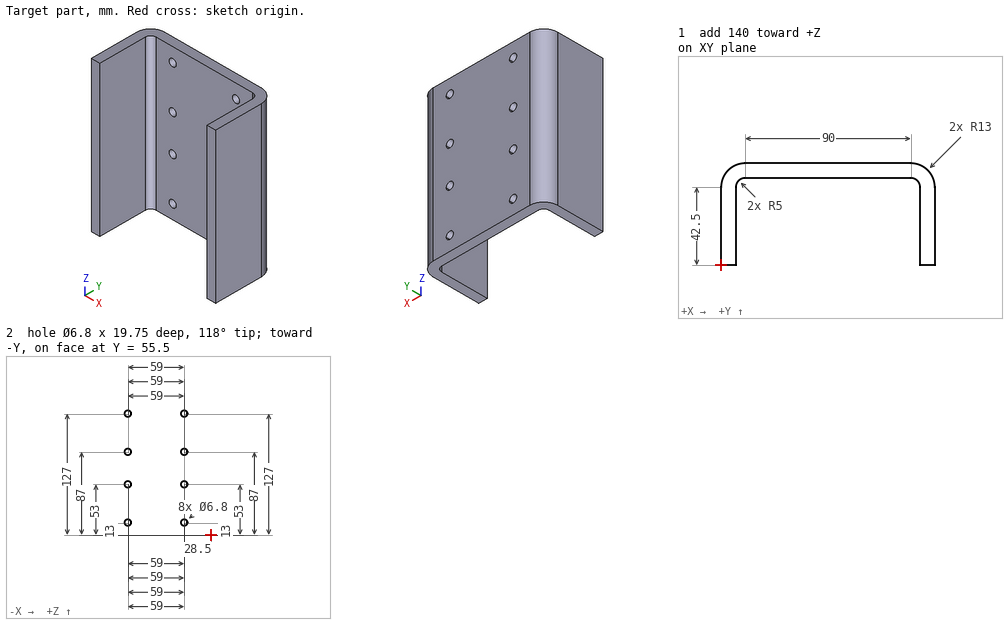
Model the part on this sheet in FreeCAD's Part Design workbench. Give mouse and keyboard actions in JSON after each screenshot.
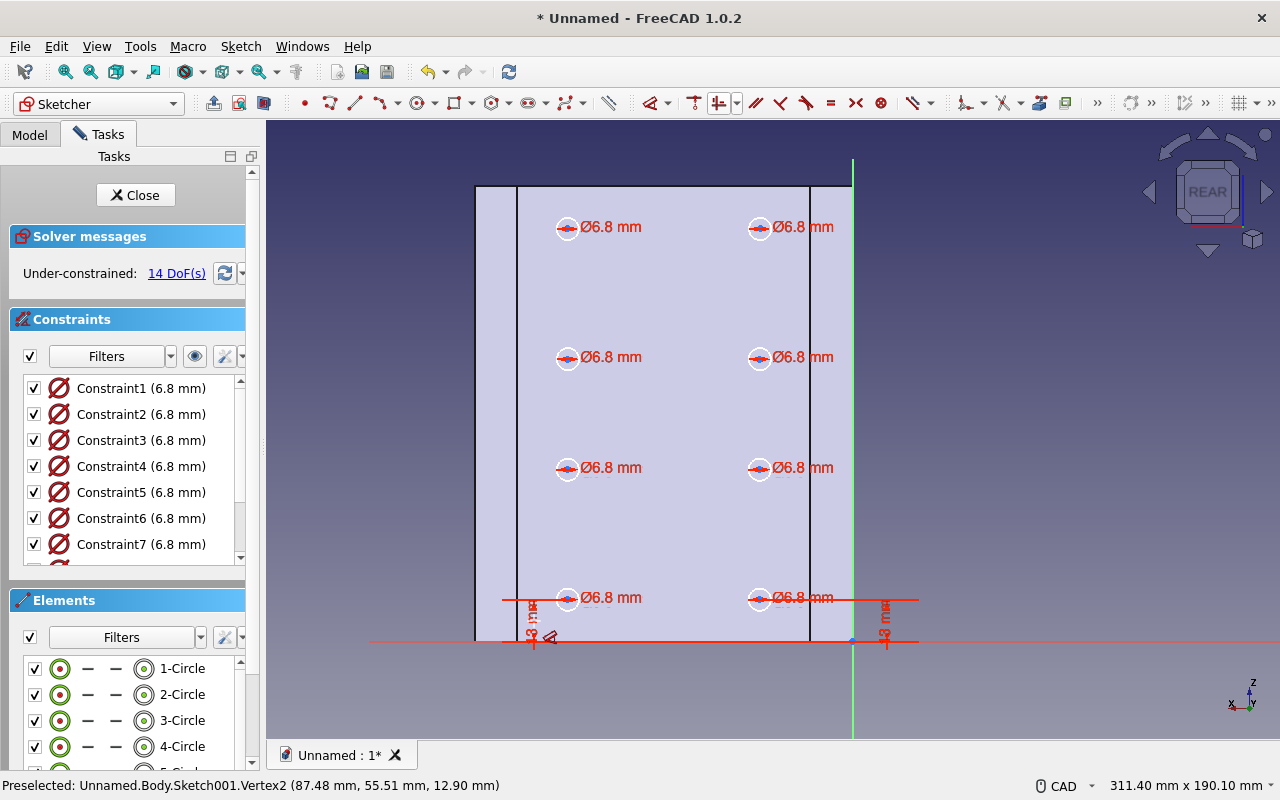
{"action": "left_click", "coordinate": [568, 470]}
{"action": "left_click", "coordinate": [887, 556]}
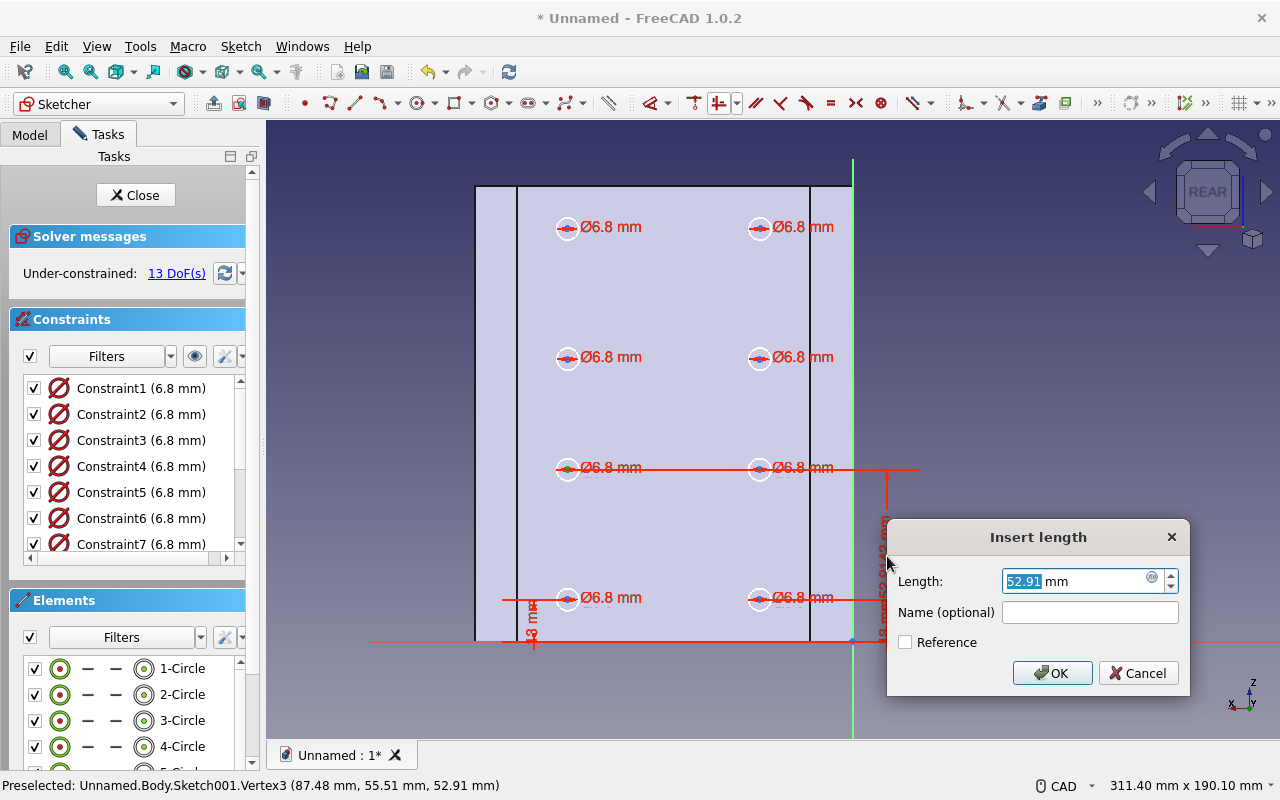
{"action": "type", "text": "53"}
{"action": "key", "text": "Return"}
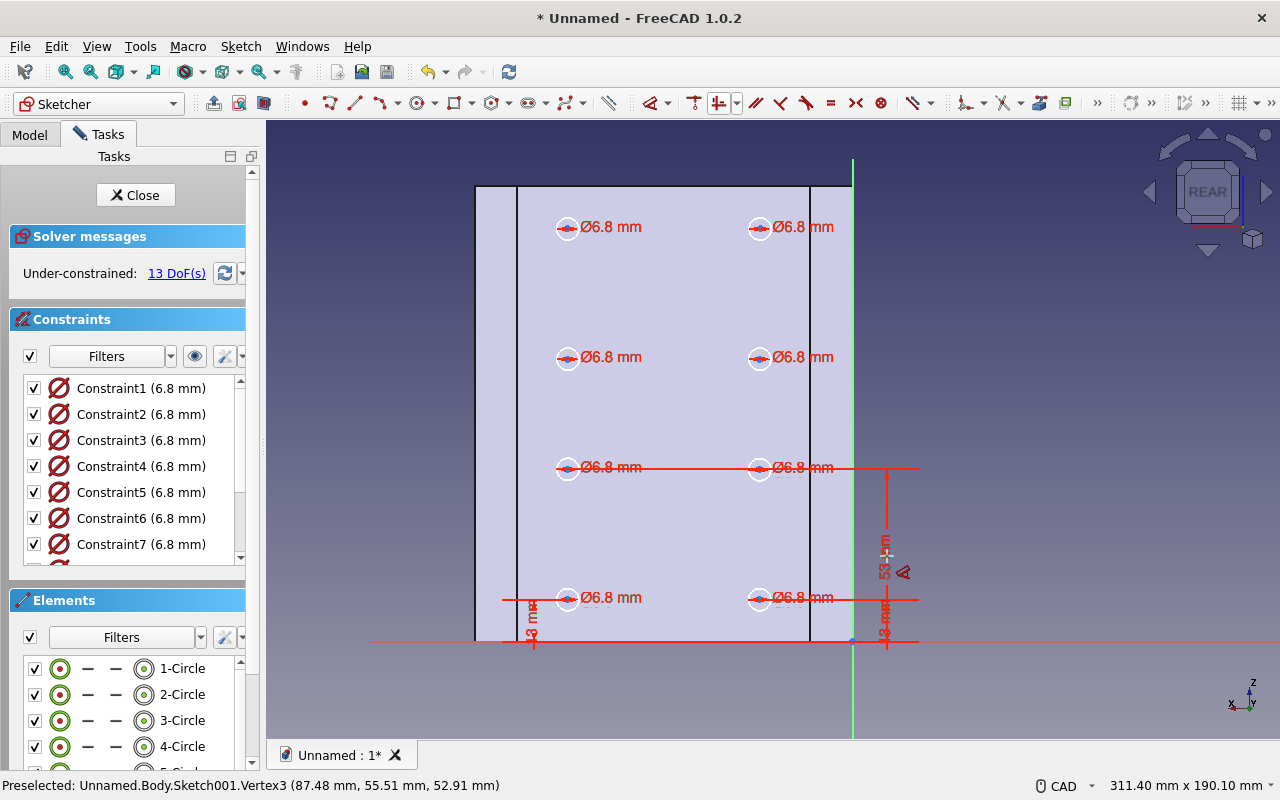
{"action": "left_click", "coordinate": [760, 470]}
{"action": "left_click", "coordinate": [887, 516]}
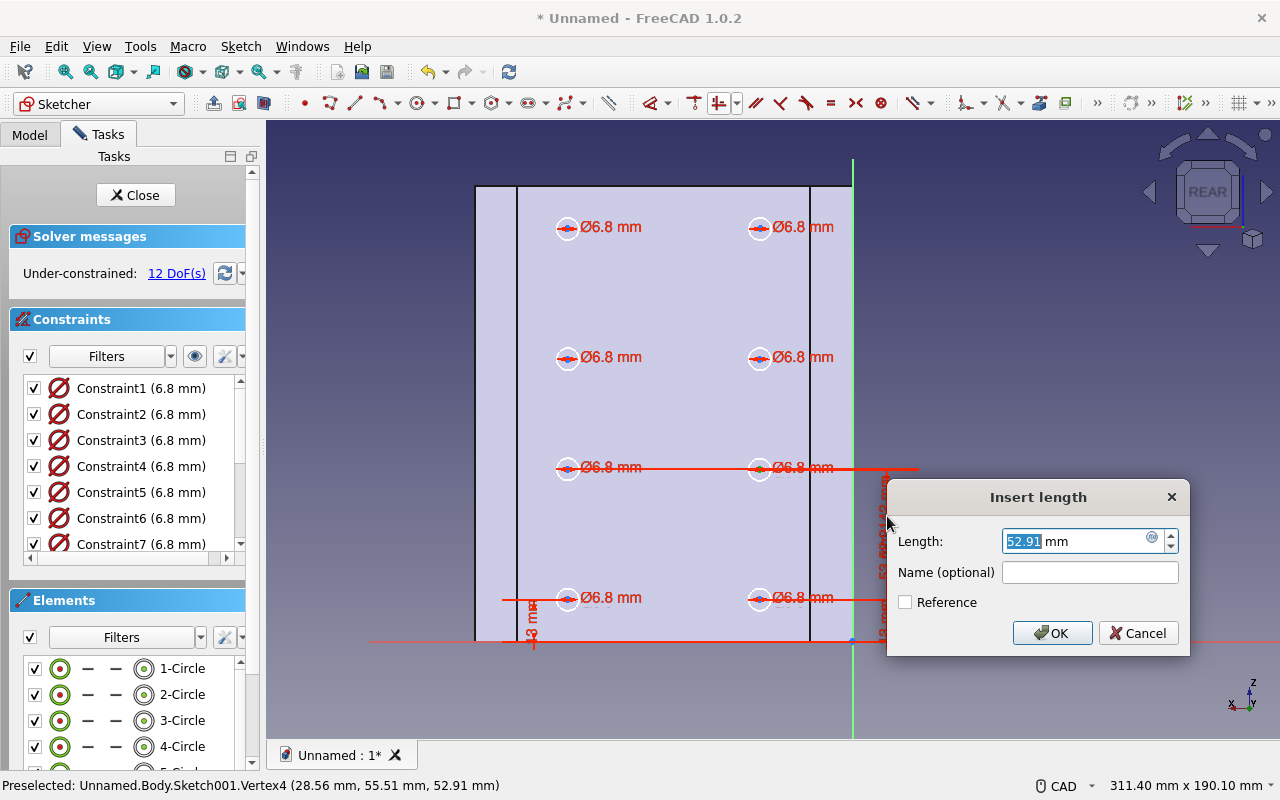
{"action": "type", "text": "53"}
{"action": "key", "text": "Return"}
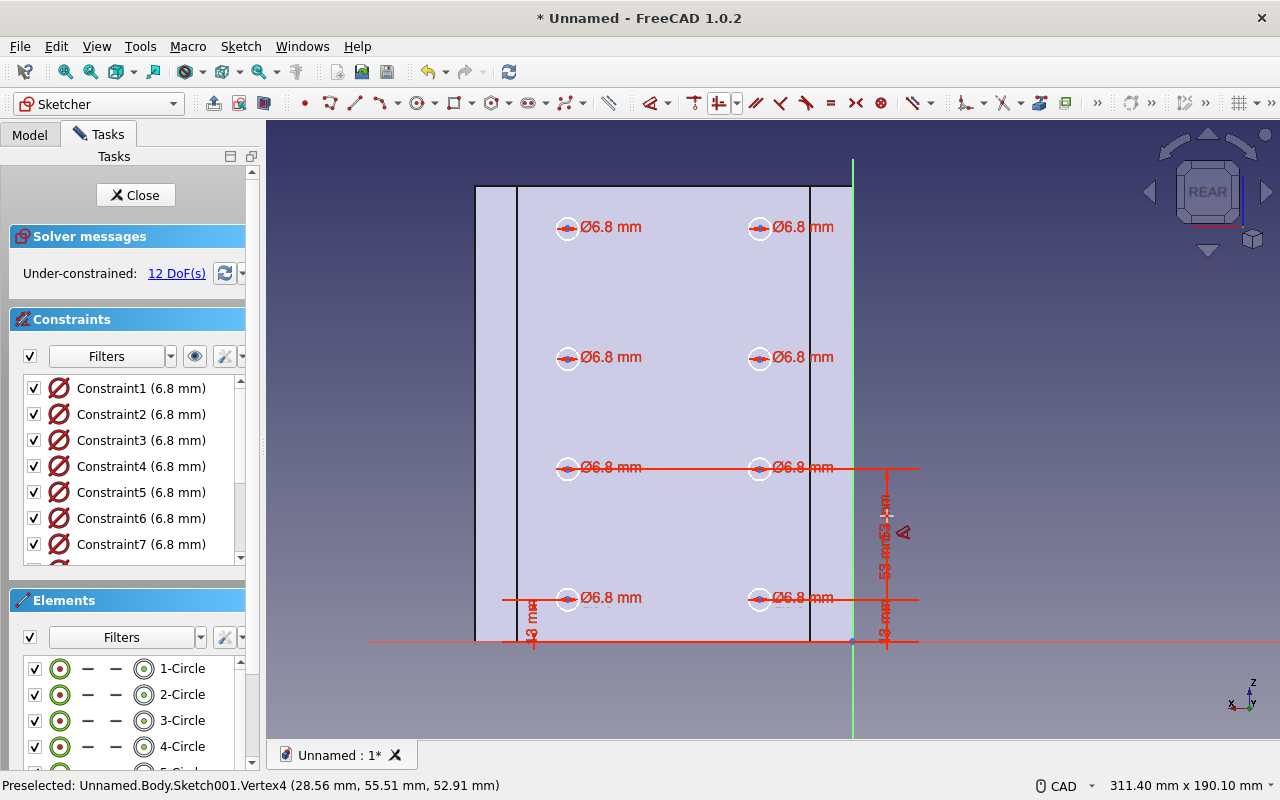
{"action": "left_click", "coordinate": [760, 359]}
{"action": "left_click", "coordinate": [887, 436]}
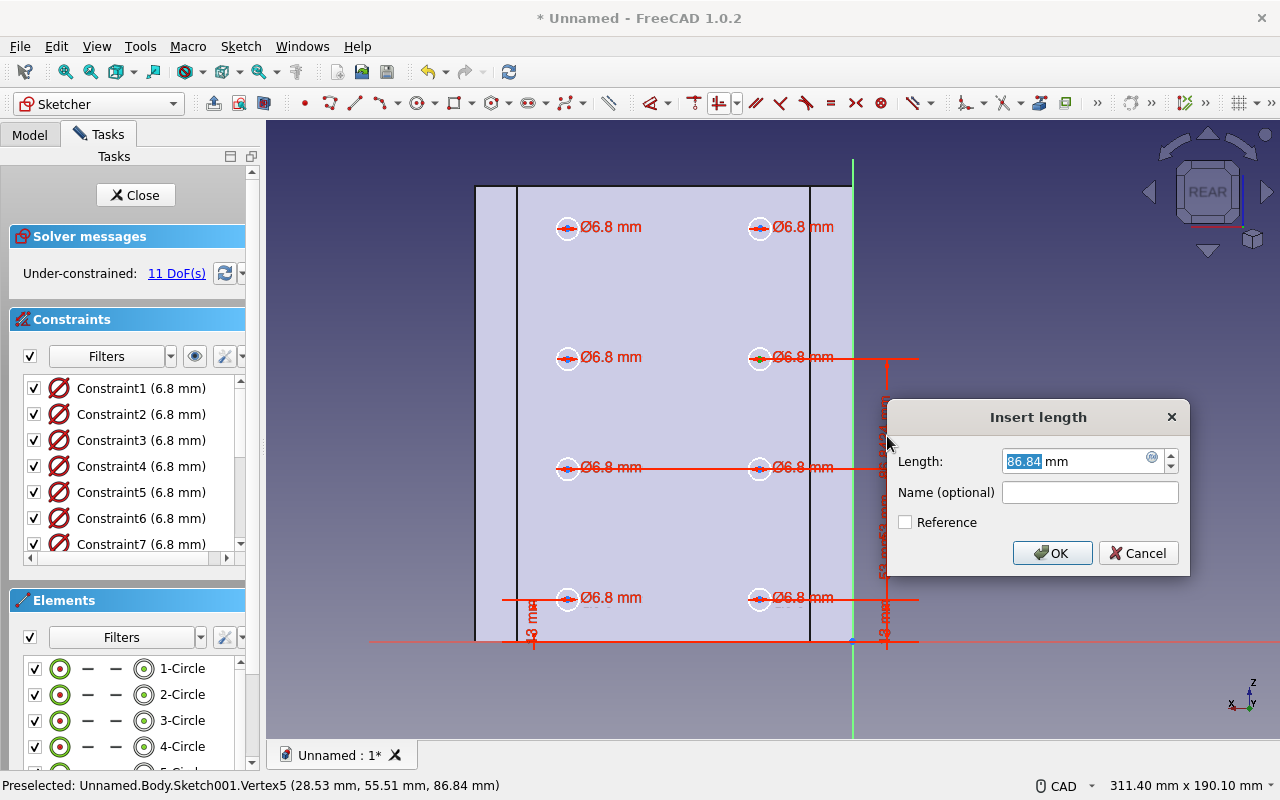
{"action": "type", "text": "87"}
{"action": "key", "text": "Return"}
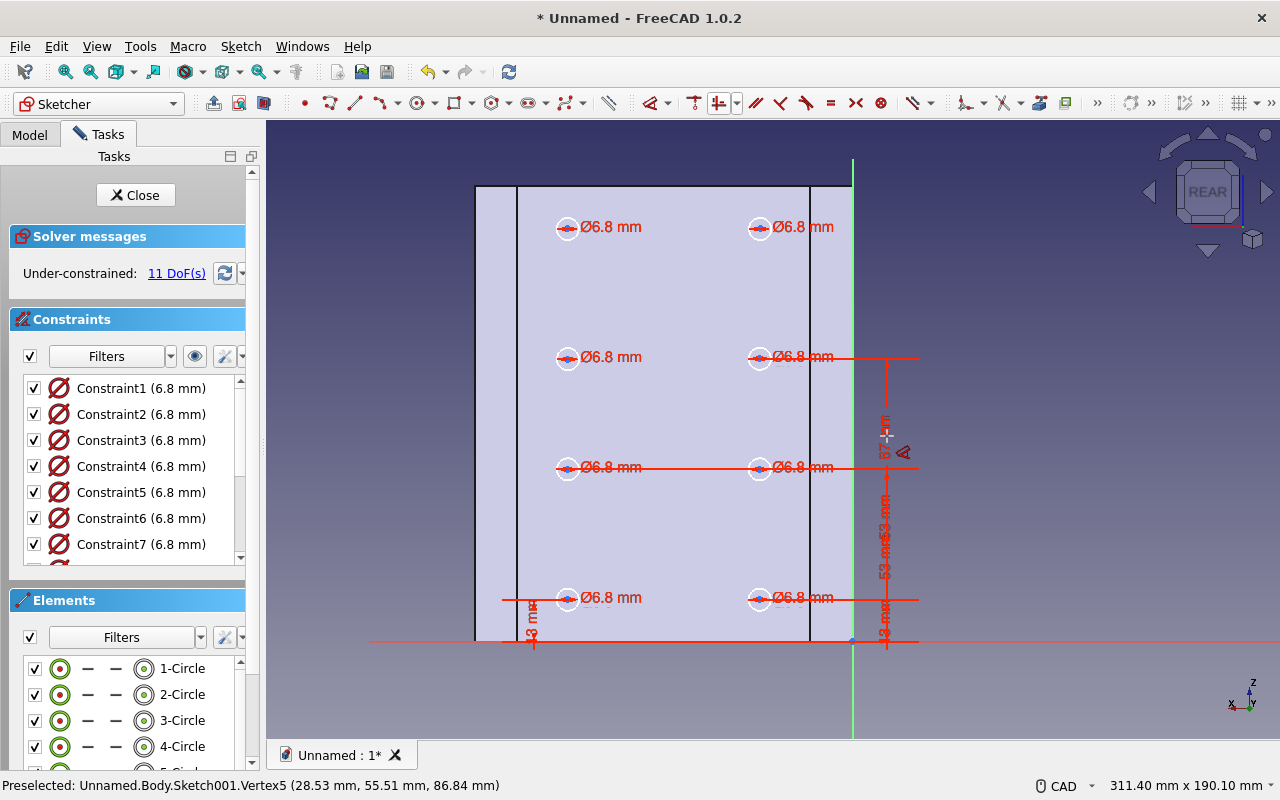
{"action": "left_click", "coordinate": [568, 359]}
{"action": "left_click", "coordinate": [887, 402]}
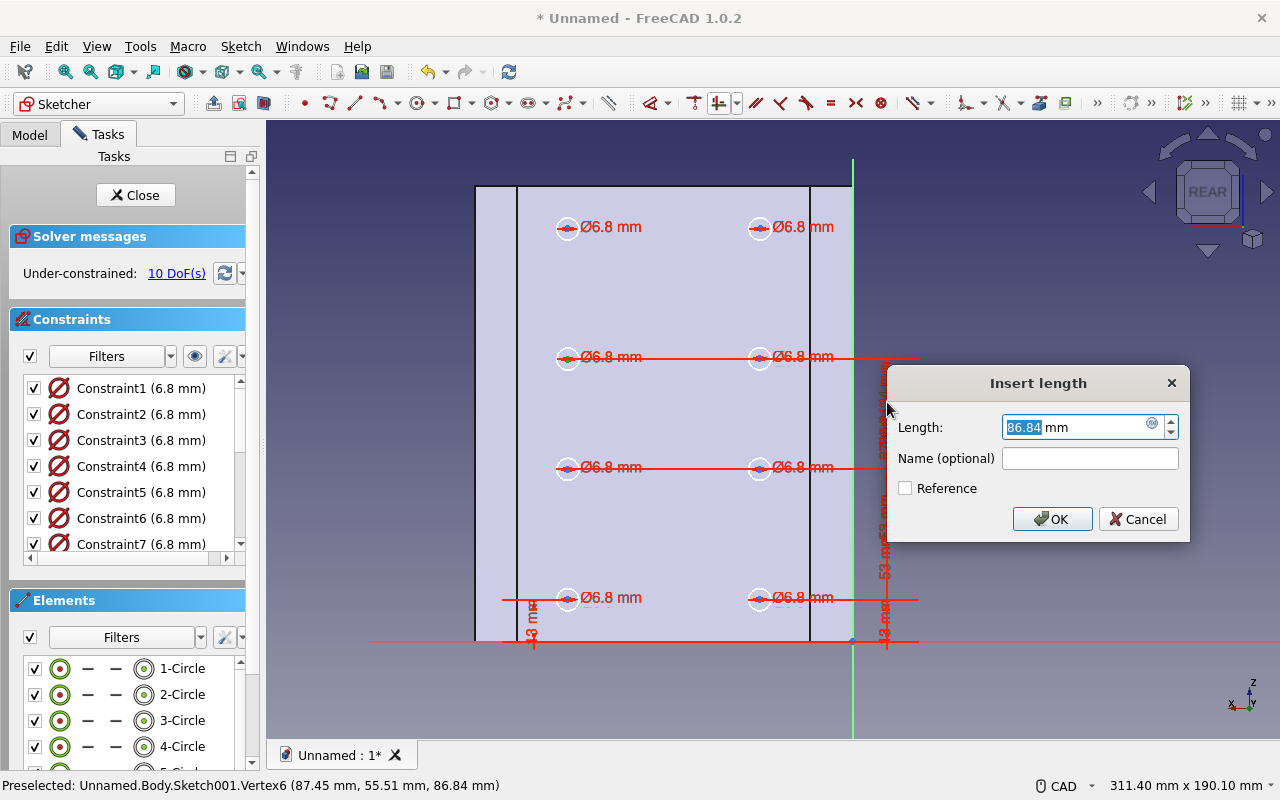
{"action": "type", "text": "87"}
{"action": "key", "text": "Return"}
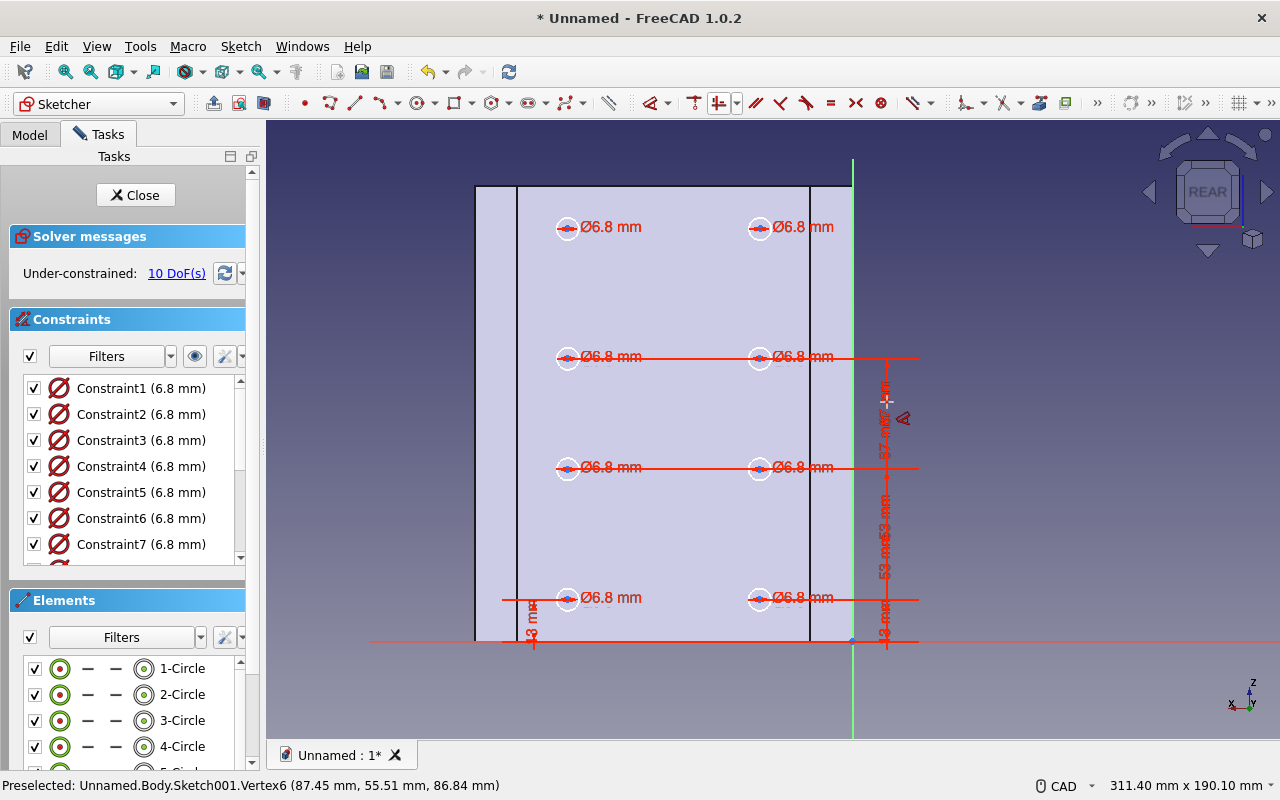
{"action": "left_click", "coordinate": [568, 229]}
{"action": "left_click", "coordinate": [887, 341]}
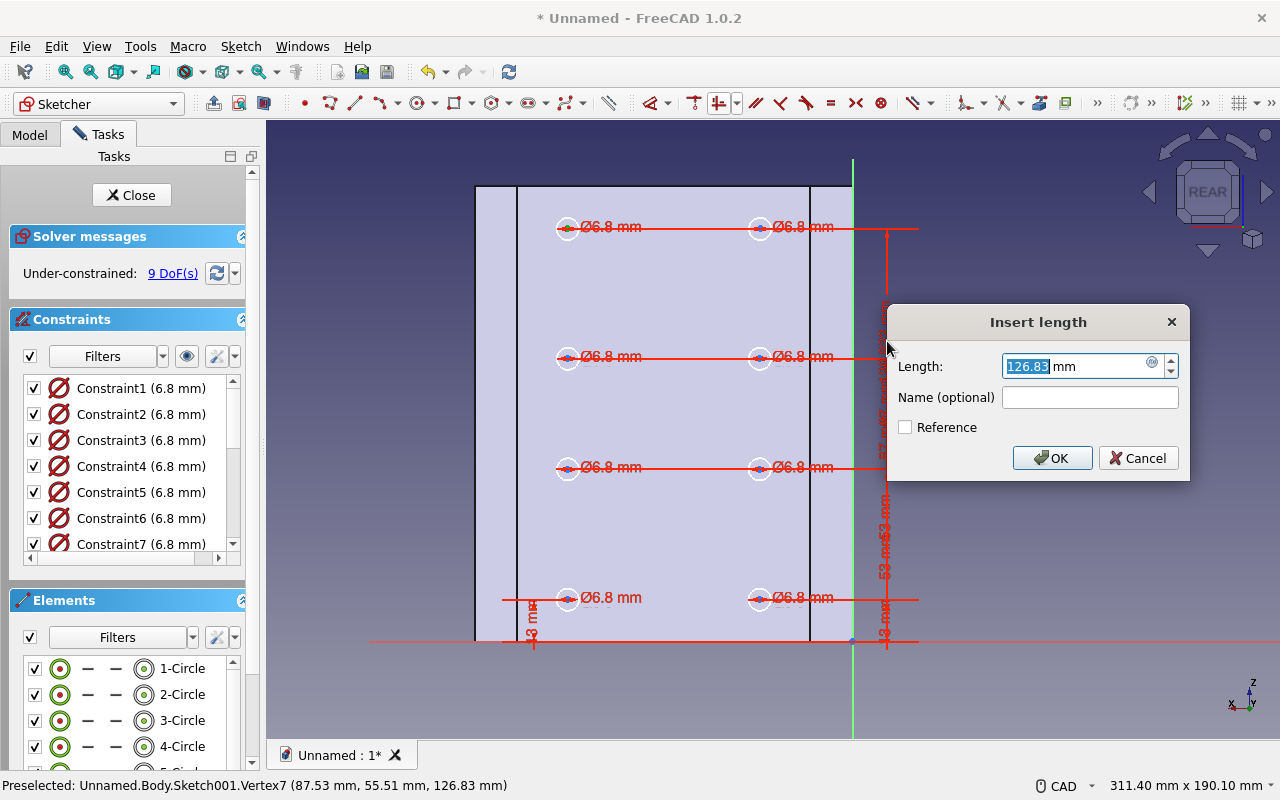
{"action": "type", "text": "127"}
{"action": "key", "text": "Return"}